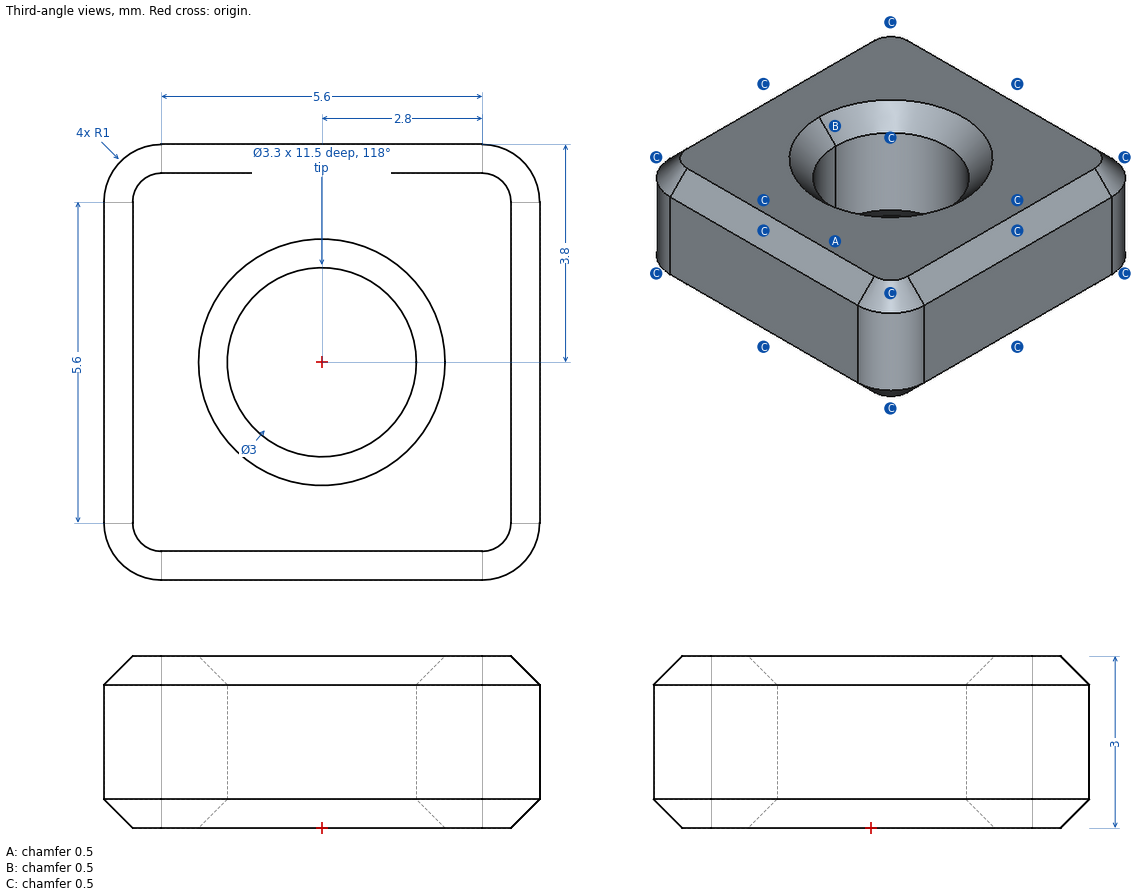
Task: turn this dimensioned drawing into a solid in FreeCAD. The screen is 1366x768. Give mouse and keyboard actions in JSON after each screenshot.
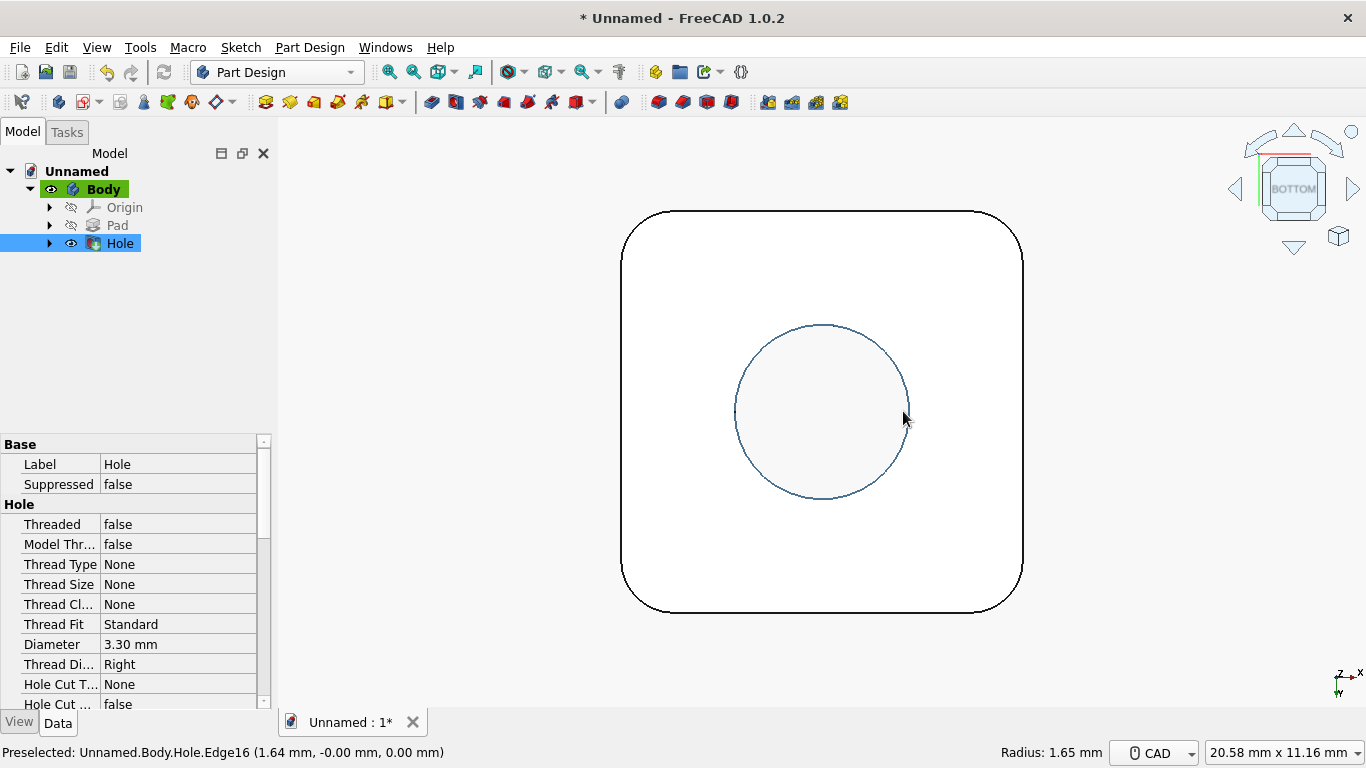
{"action": "left_click", "coordinate": [684, 102]}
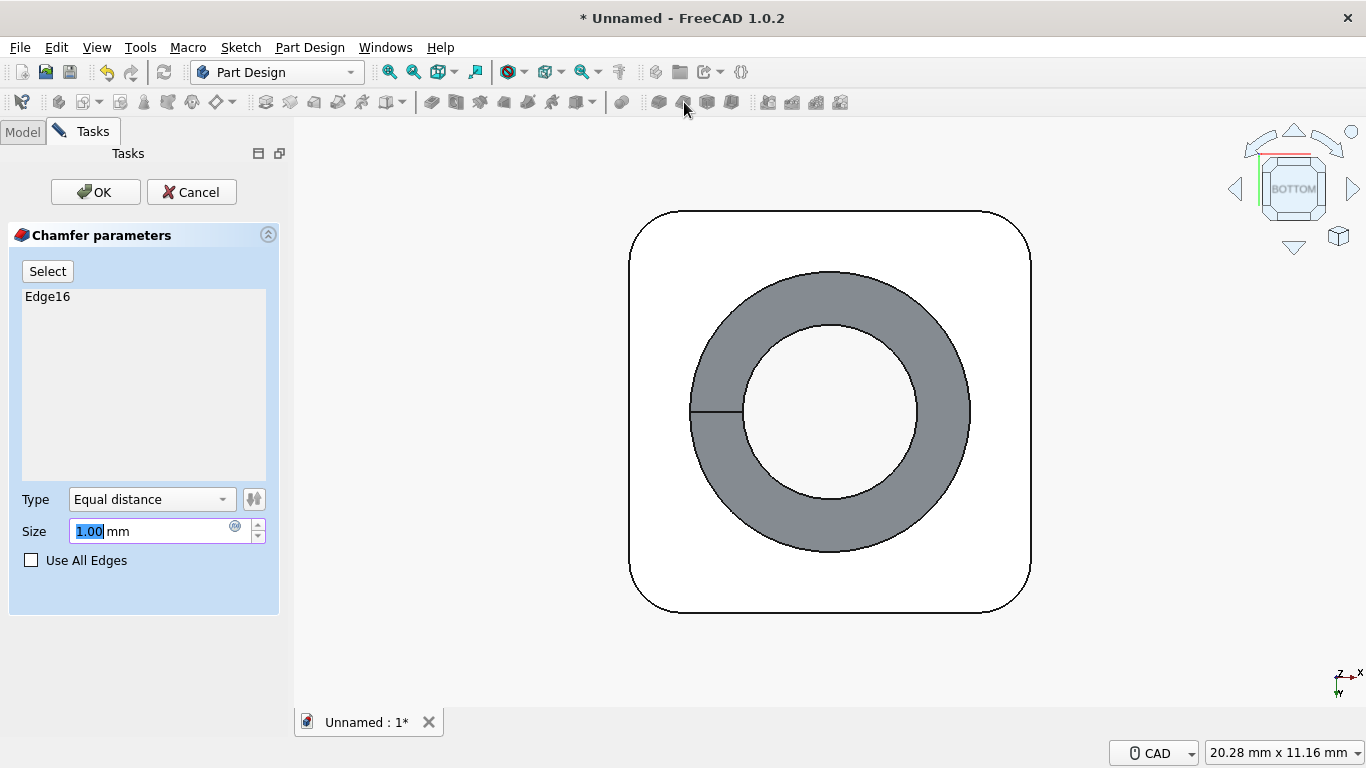
{"action": "type", "text": "0.5"}
{"action": "key", "text": "Tab"}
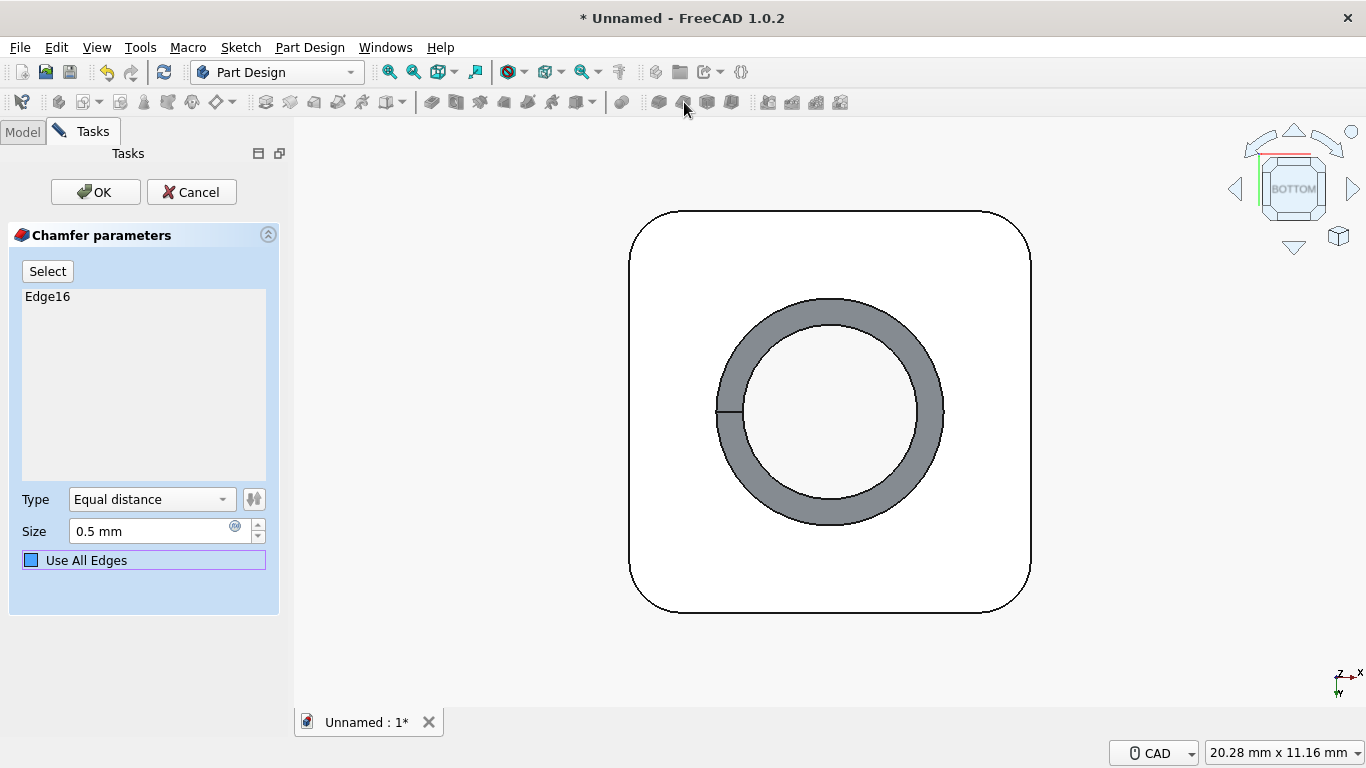
{"action": "left_click", "coordinate": [96, 192]}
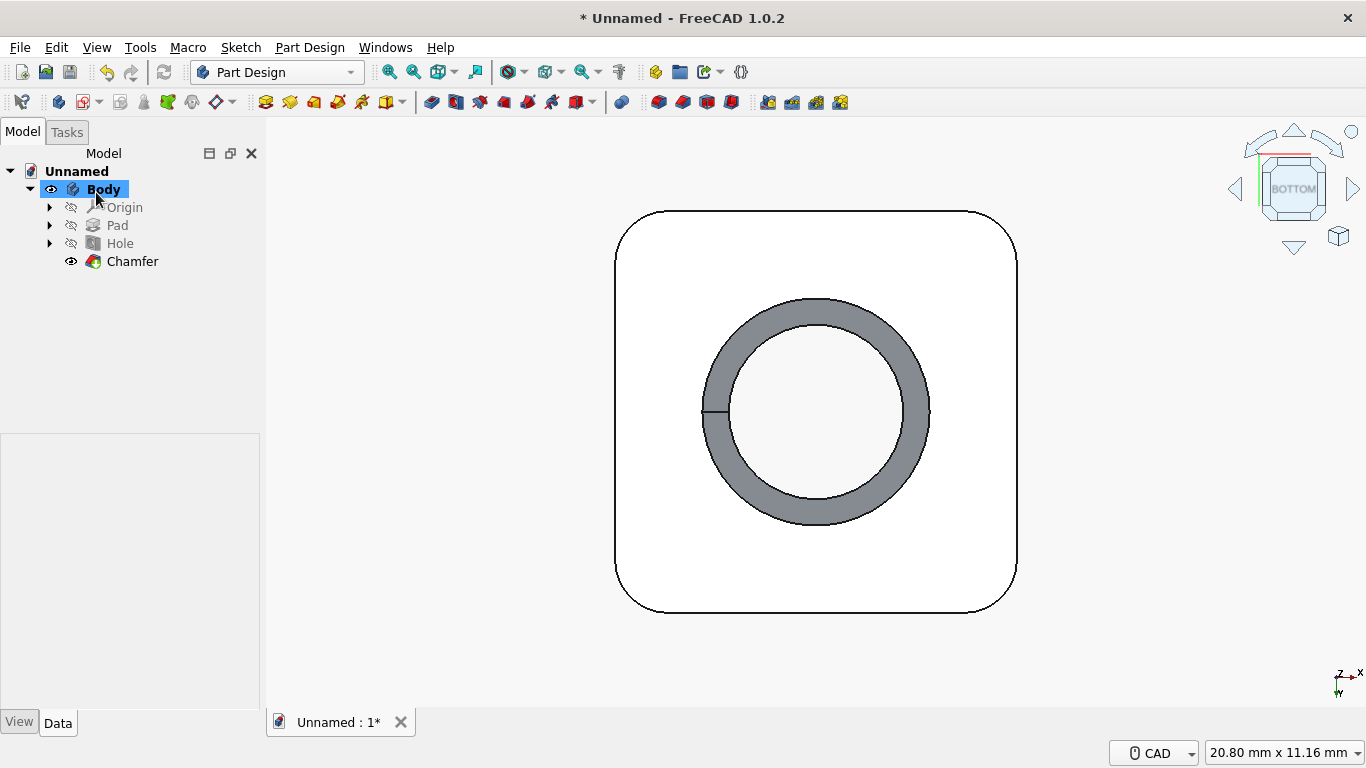
{"action": "key", "text": "0"}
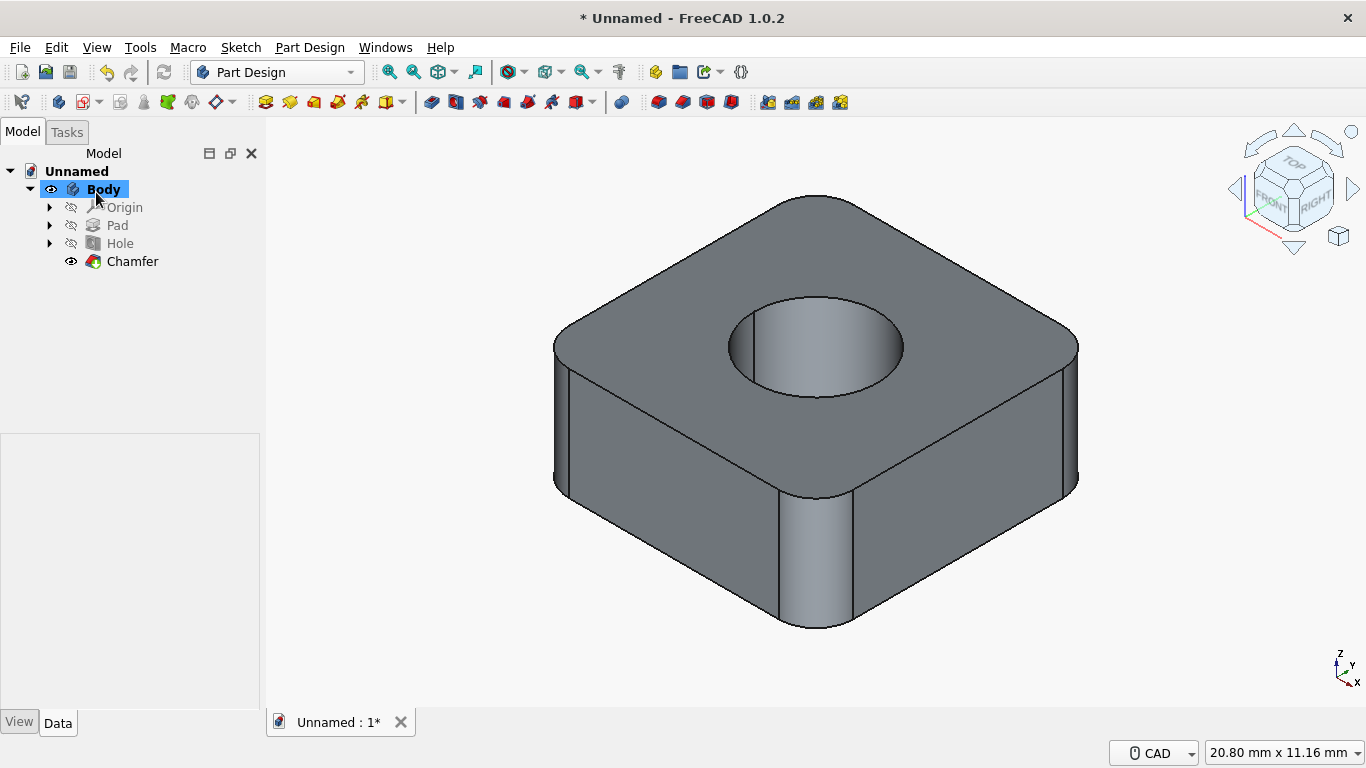
{"action": "left_click", "coordinate": [894, 323]}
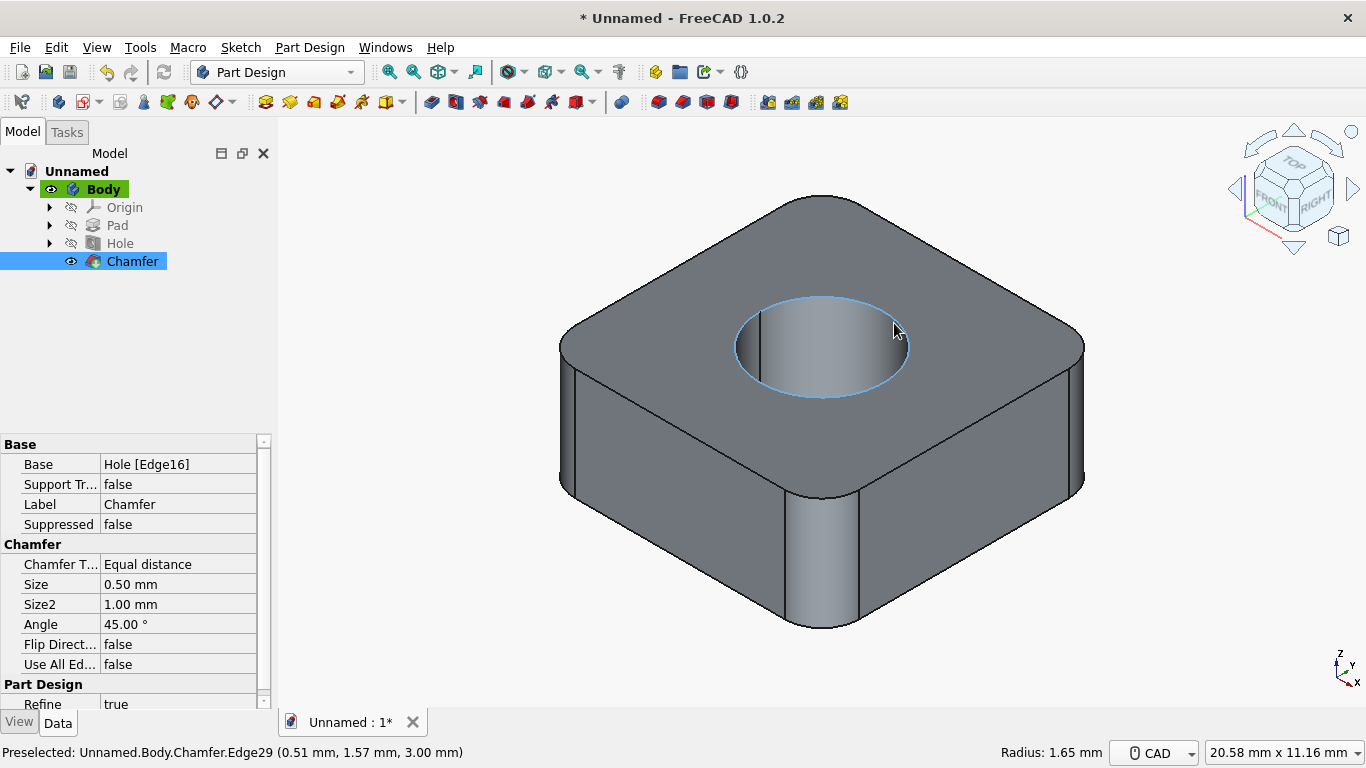
{"action": "left_click", "coordinate": [684, 102]}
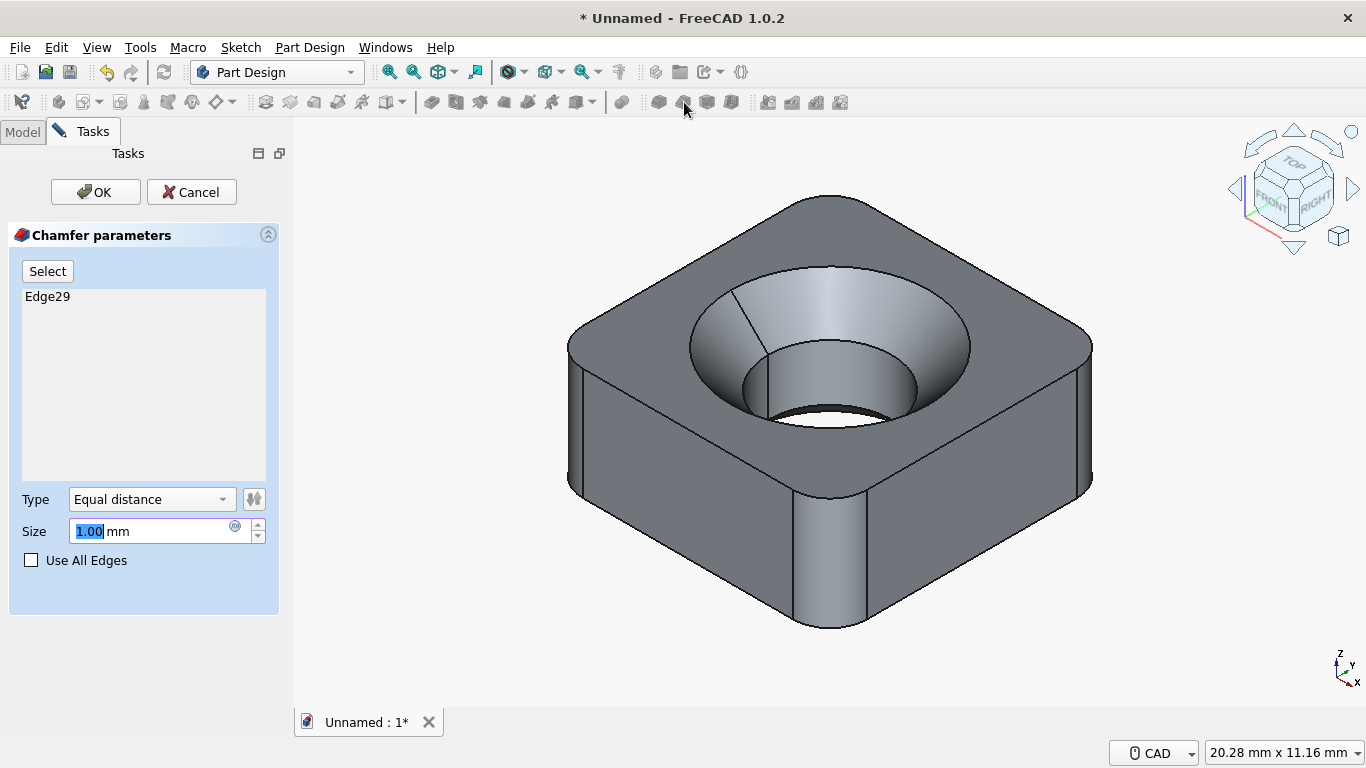
{"action": "type", "text": "0.5"}
{"action": "key", "text": "Tab"}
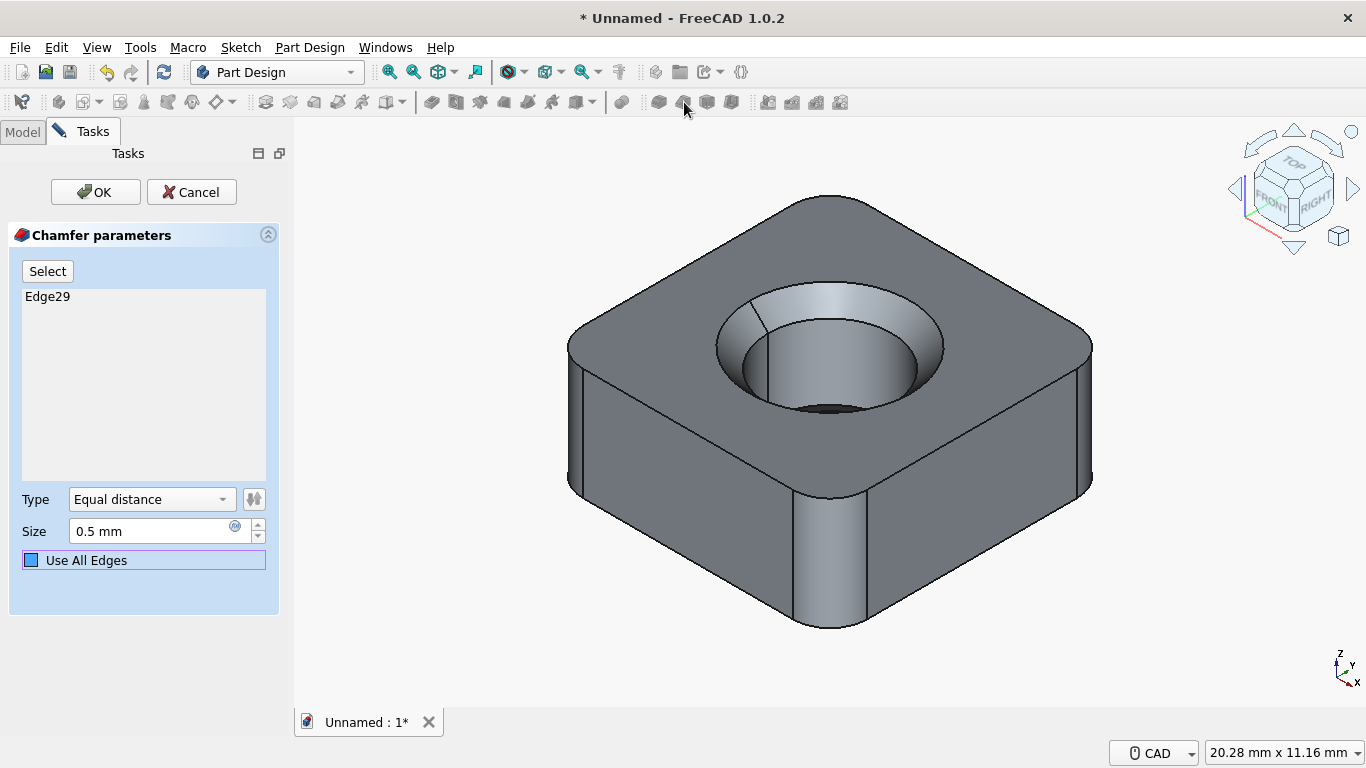
{"action": "left_click", "coordinate": [96, 192]}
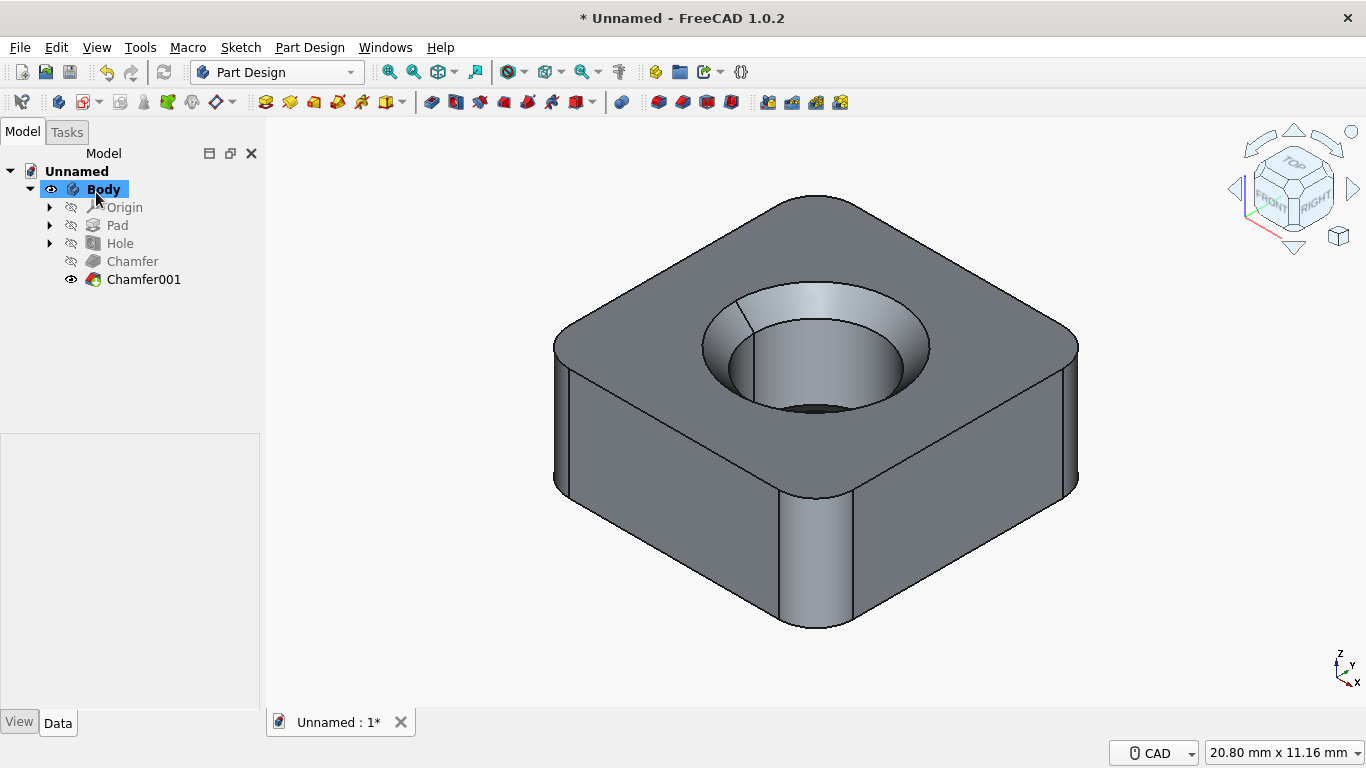
{"action": "left_click", "coordinate": [816, 498]}